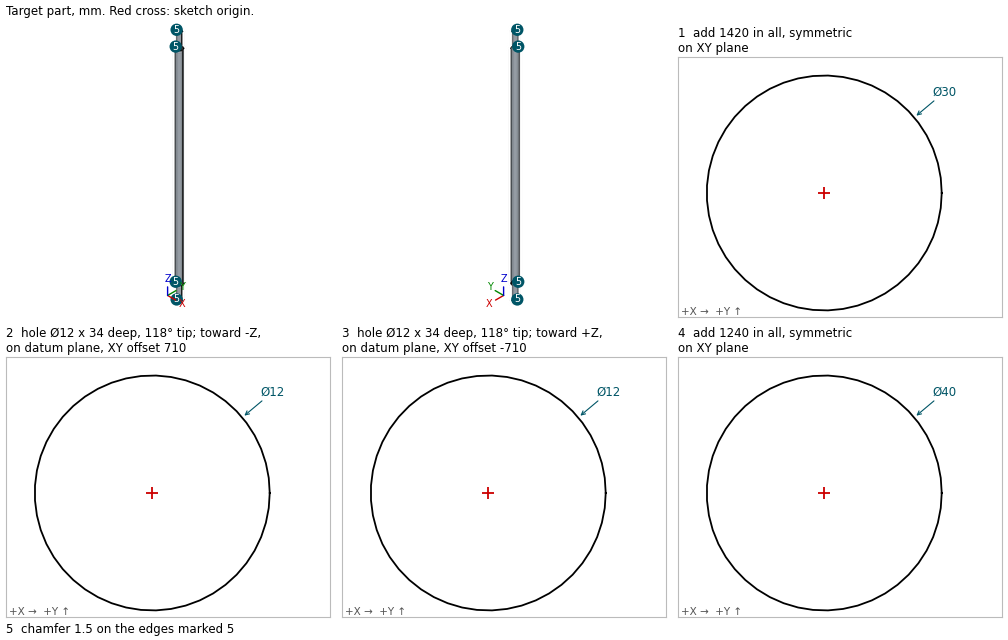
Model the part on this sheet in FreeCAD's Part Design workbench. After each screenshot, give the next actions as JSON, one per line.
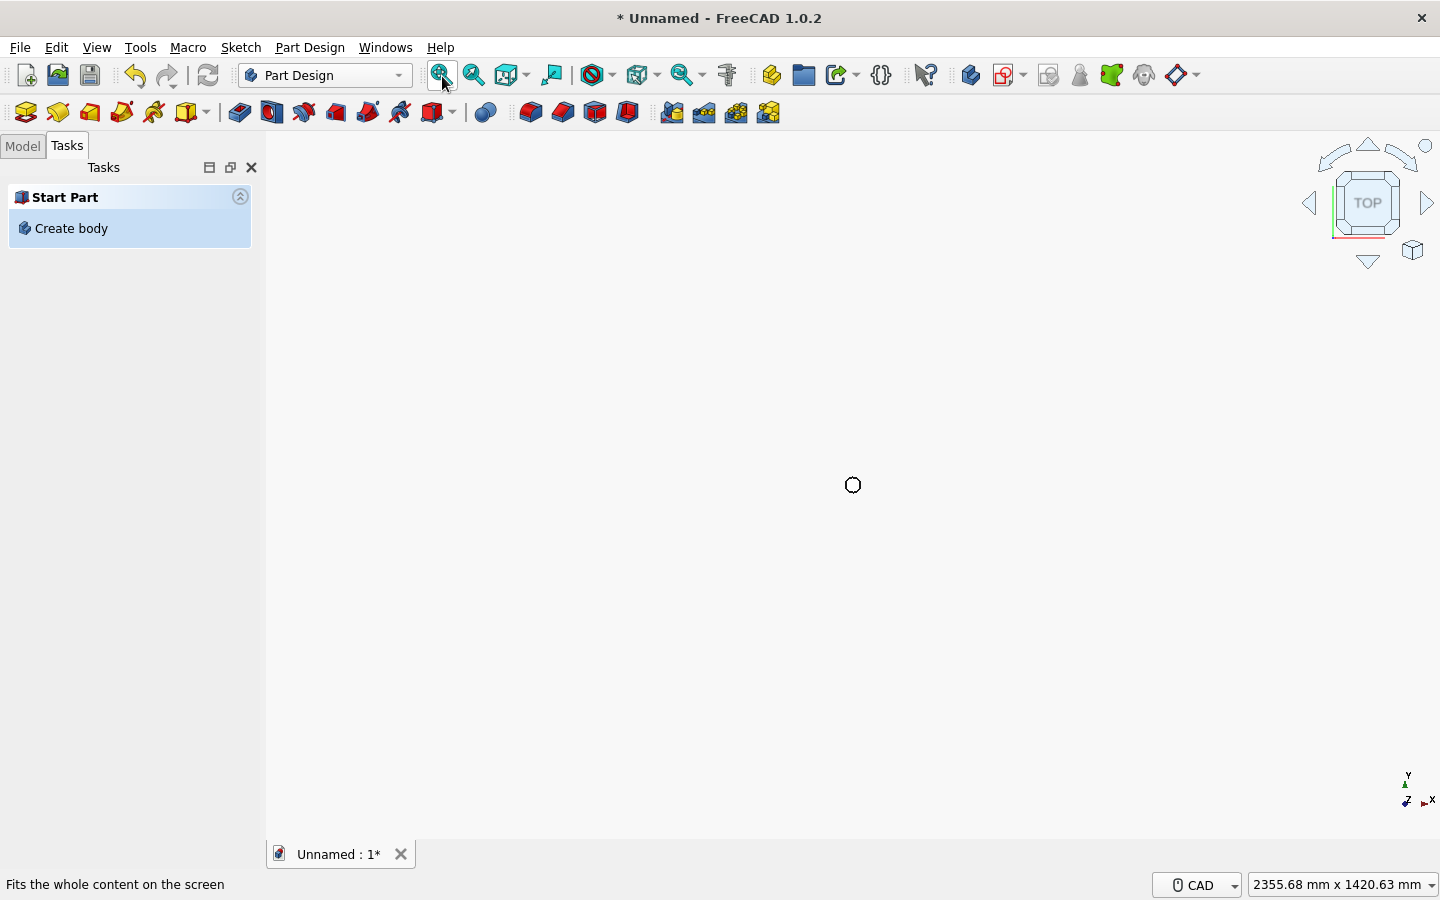
{"action": "left_click", "coordinate": [442, 76]}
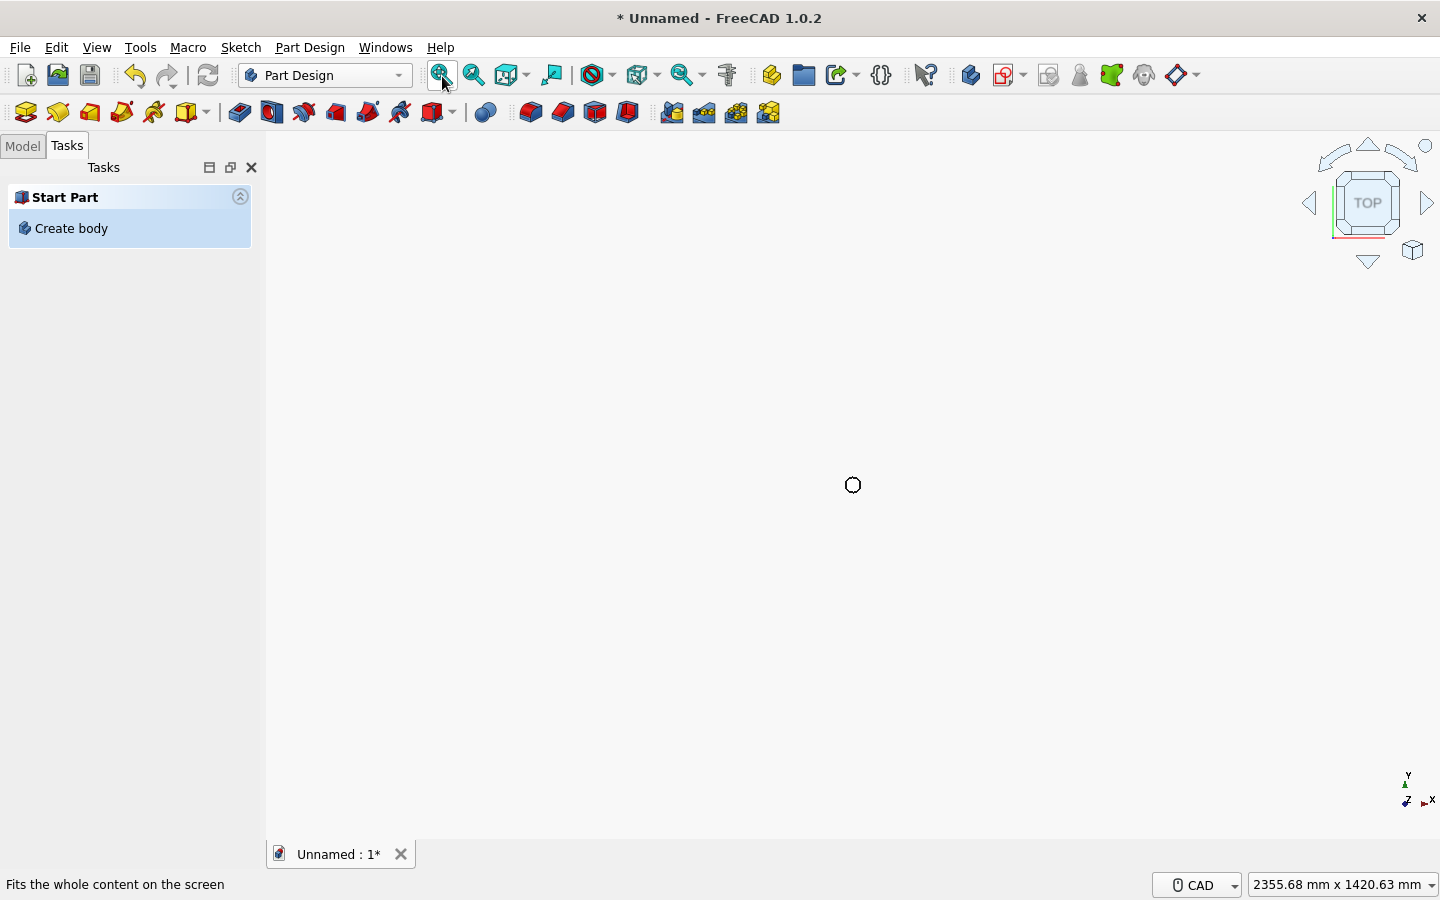
{"action": "key", "text": "1"}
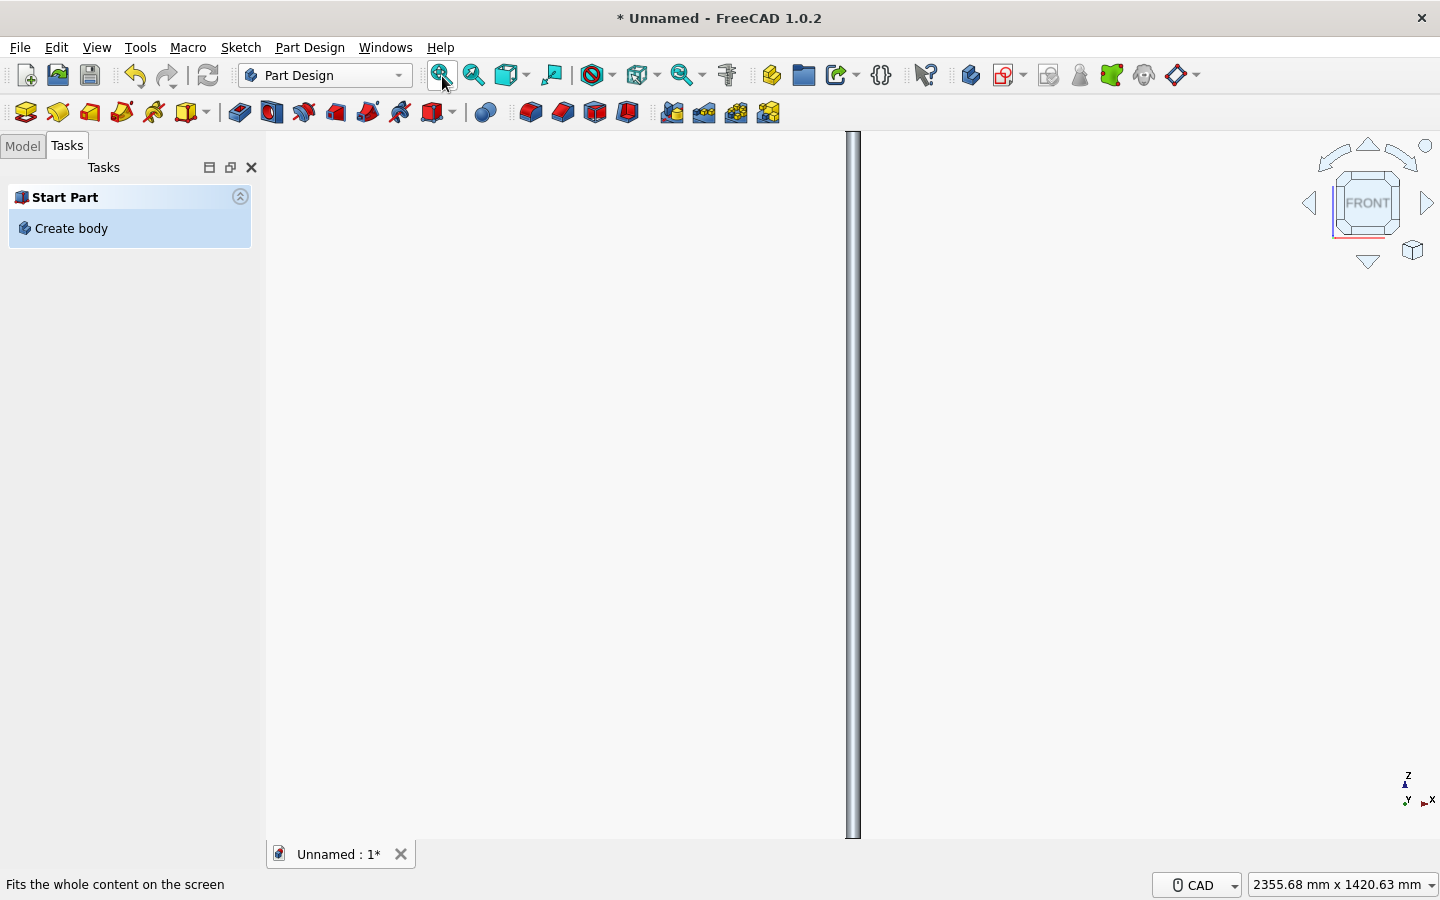
{"action": "left_click", "coordinate": [442, 76]}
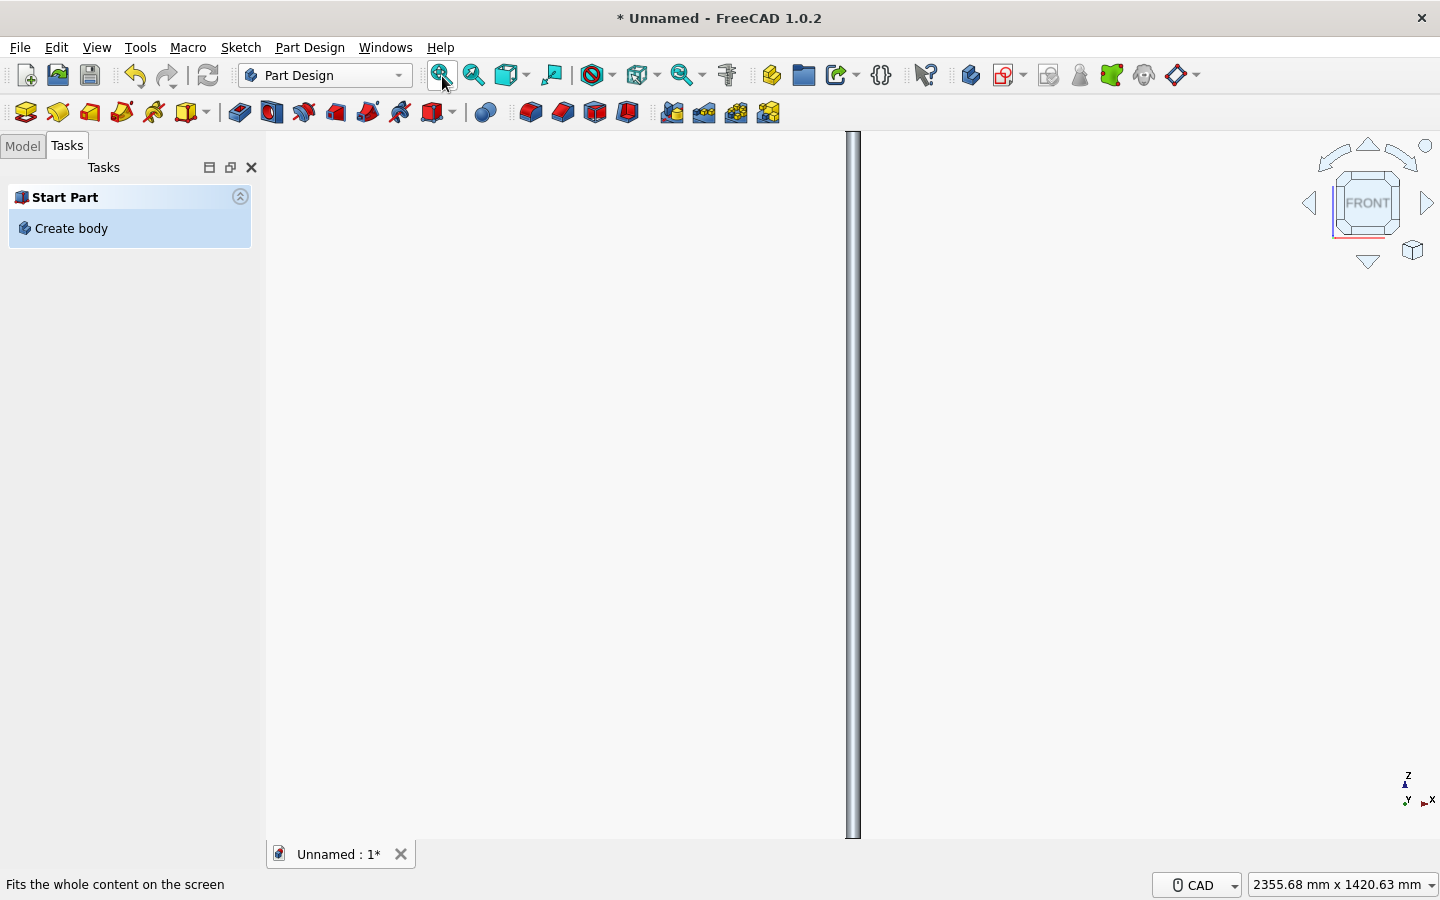
{"action": "left_click", "coordinate": [23, 145]}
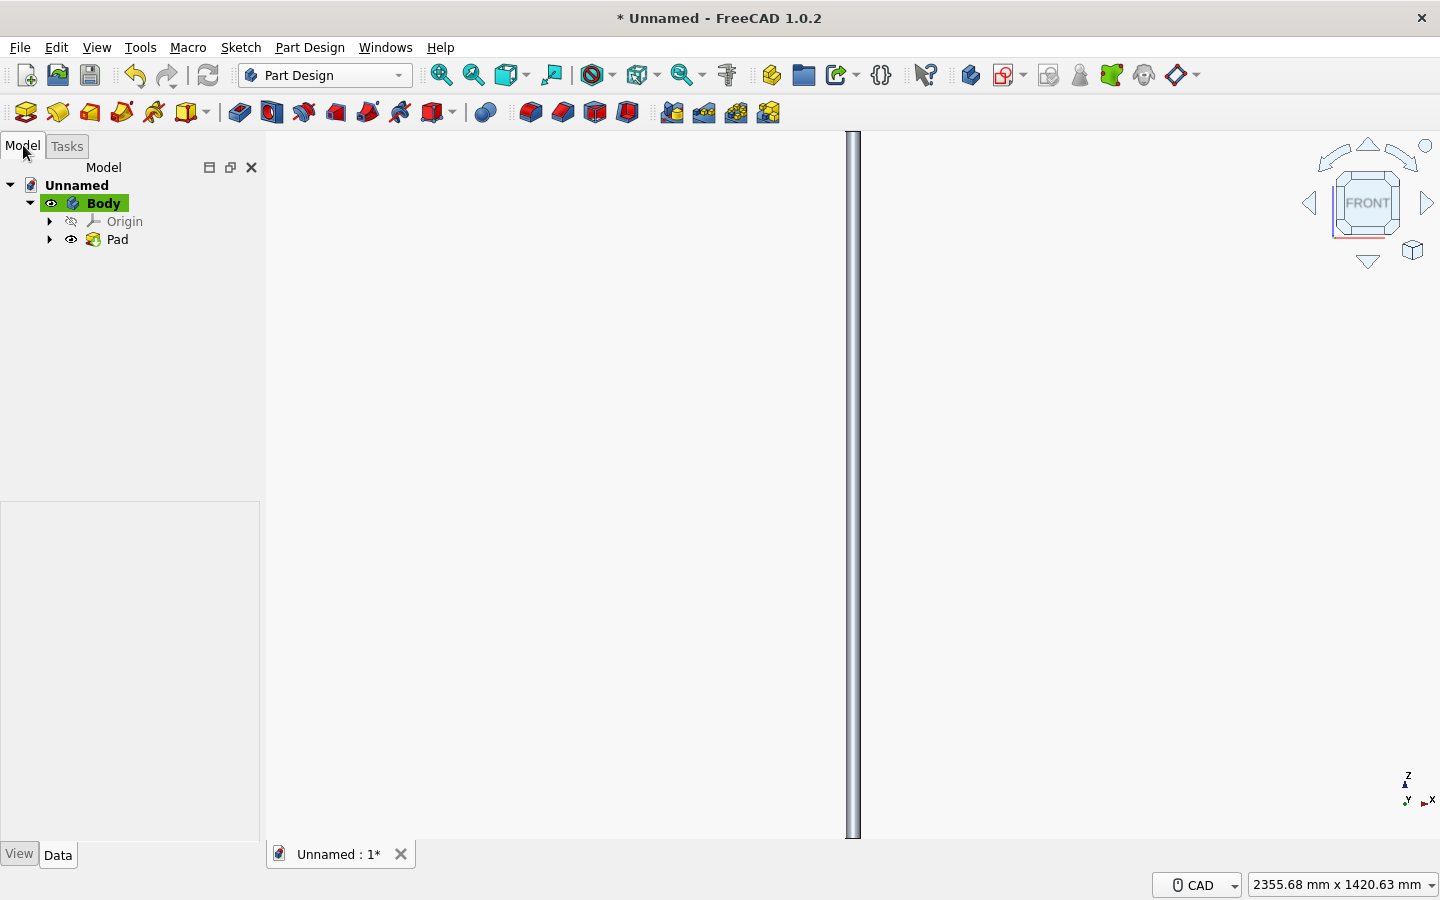
{"action": "left_click", "coordinate": [50, 221]}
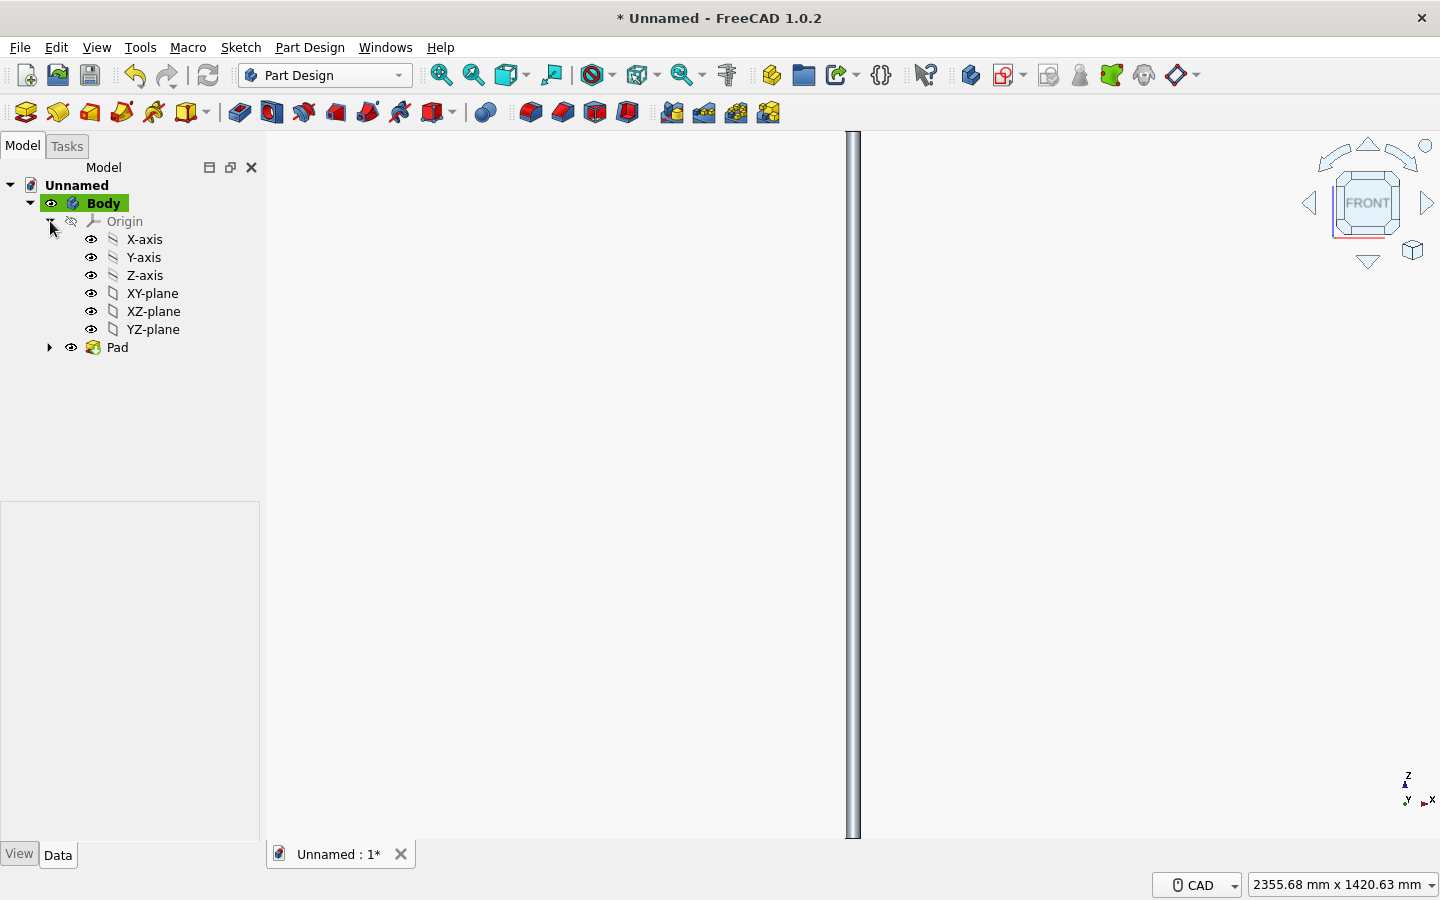
{"action": "left_click", "coordinate": [136, 293]}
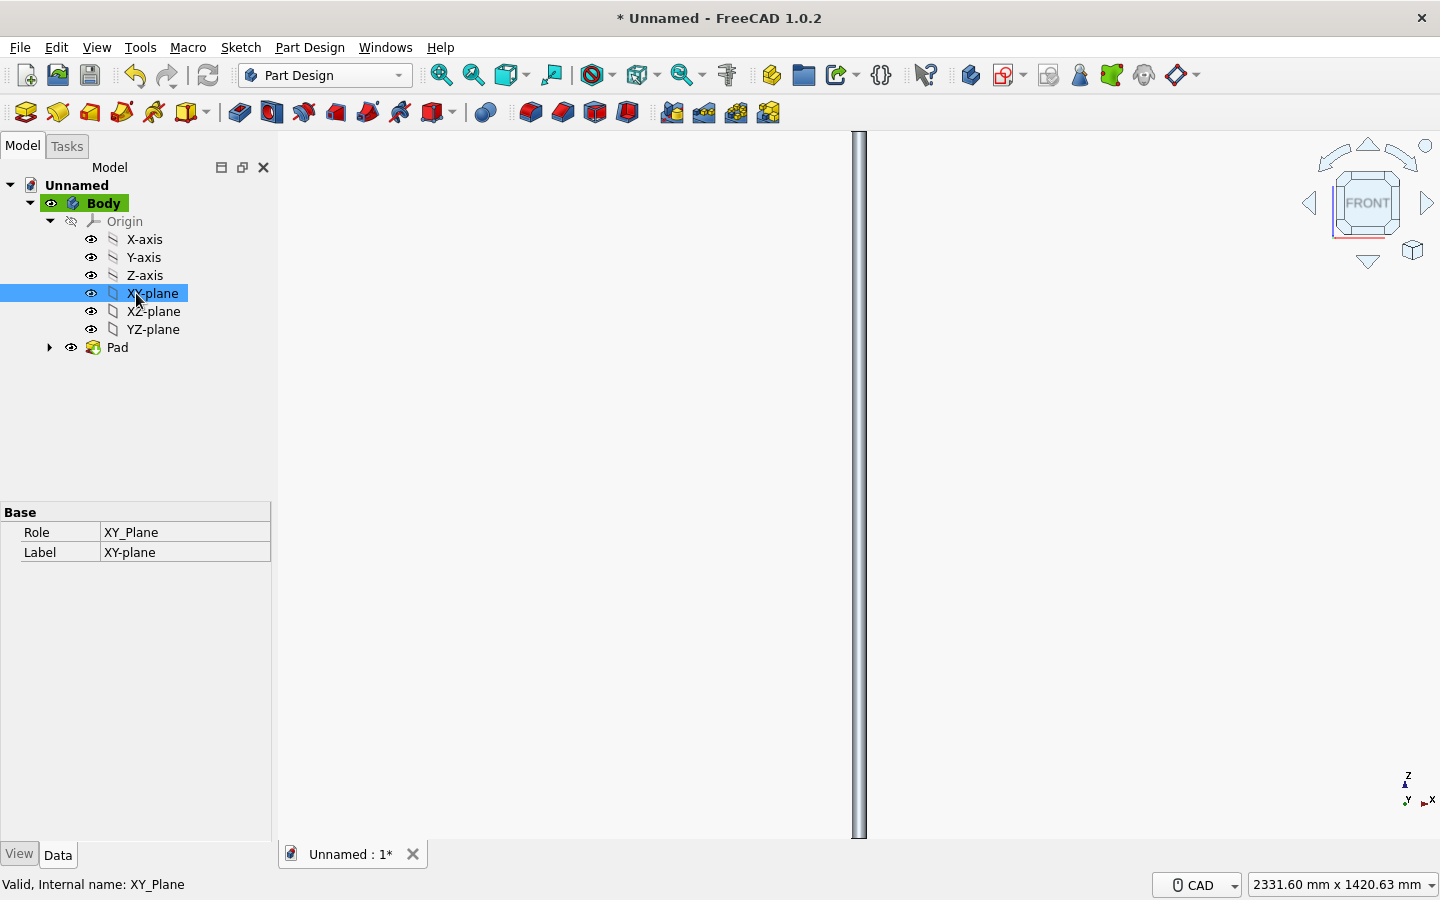
{"action": "left_click", "coordinate": [1176, 76]}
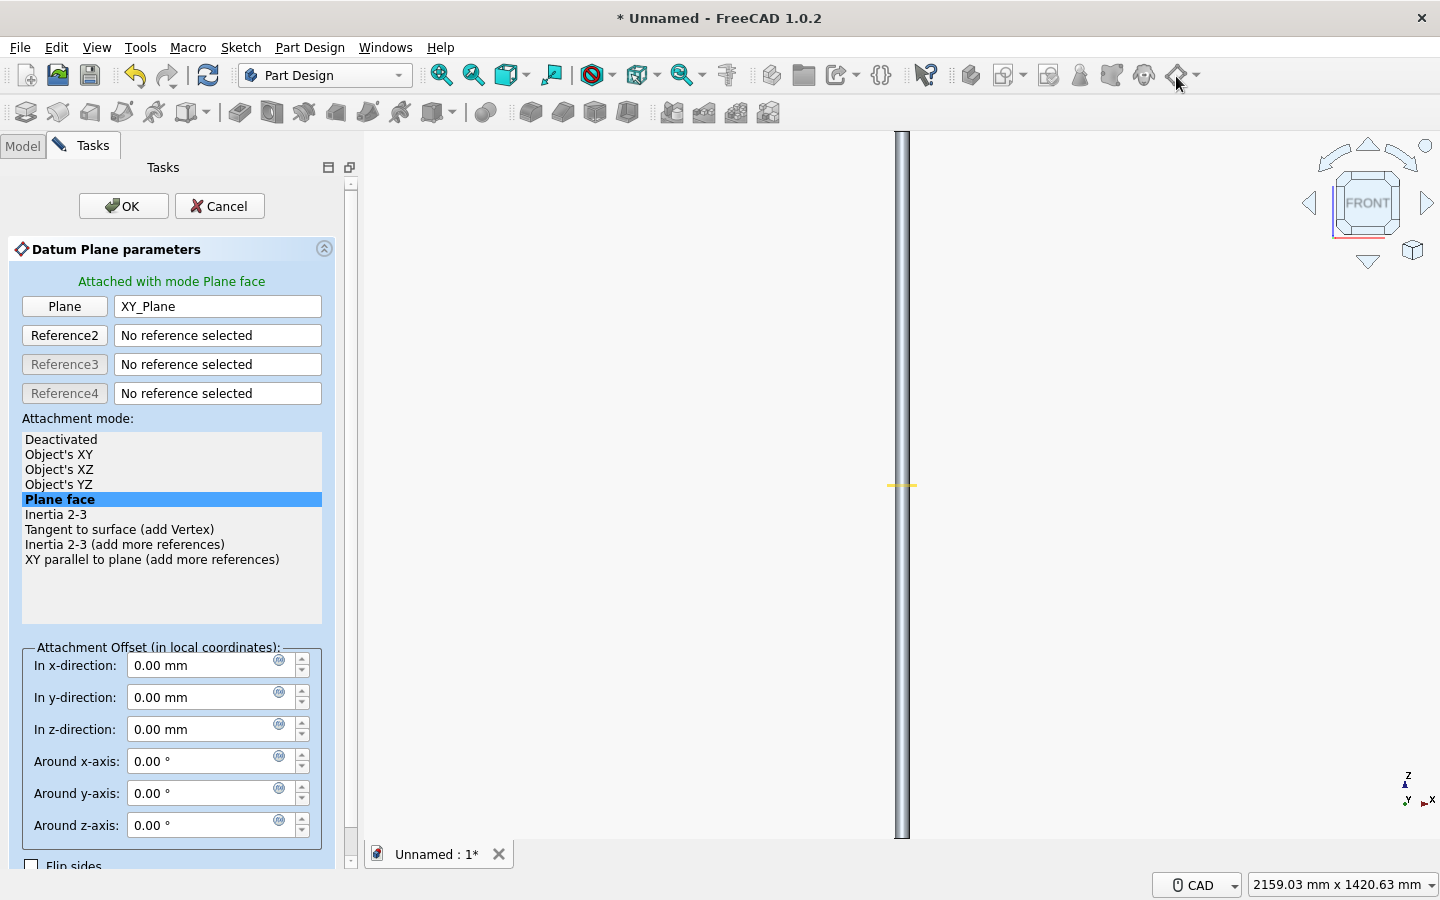
{"action": "triple_click", "coordinate": [210, 729]}